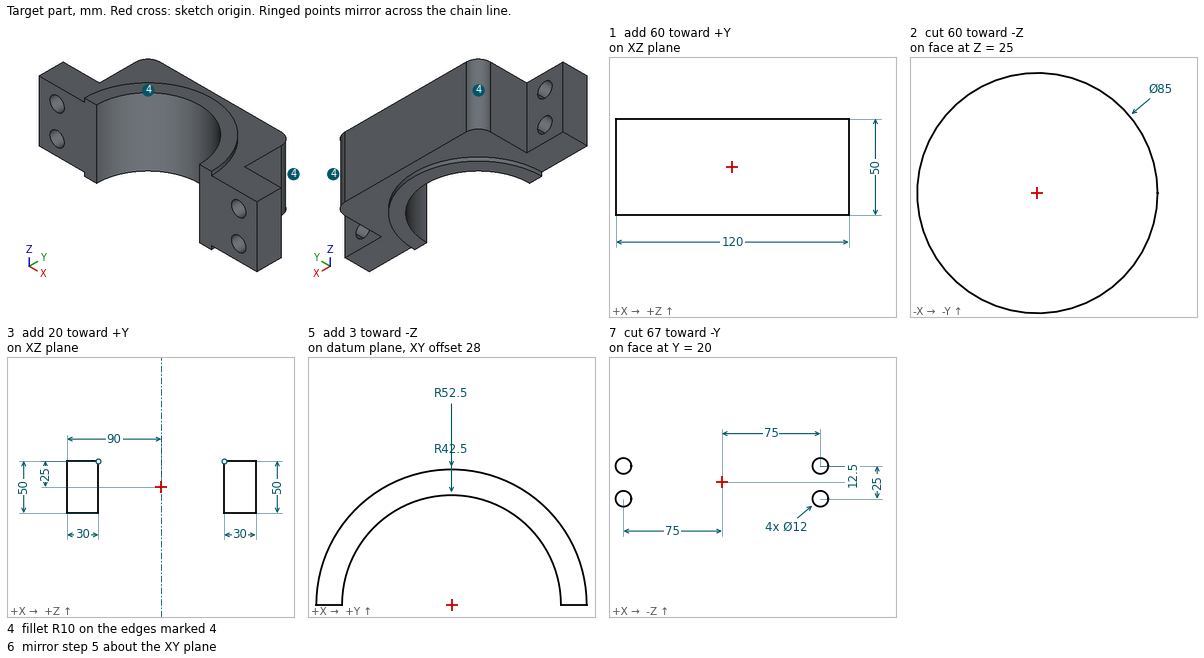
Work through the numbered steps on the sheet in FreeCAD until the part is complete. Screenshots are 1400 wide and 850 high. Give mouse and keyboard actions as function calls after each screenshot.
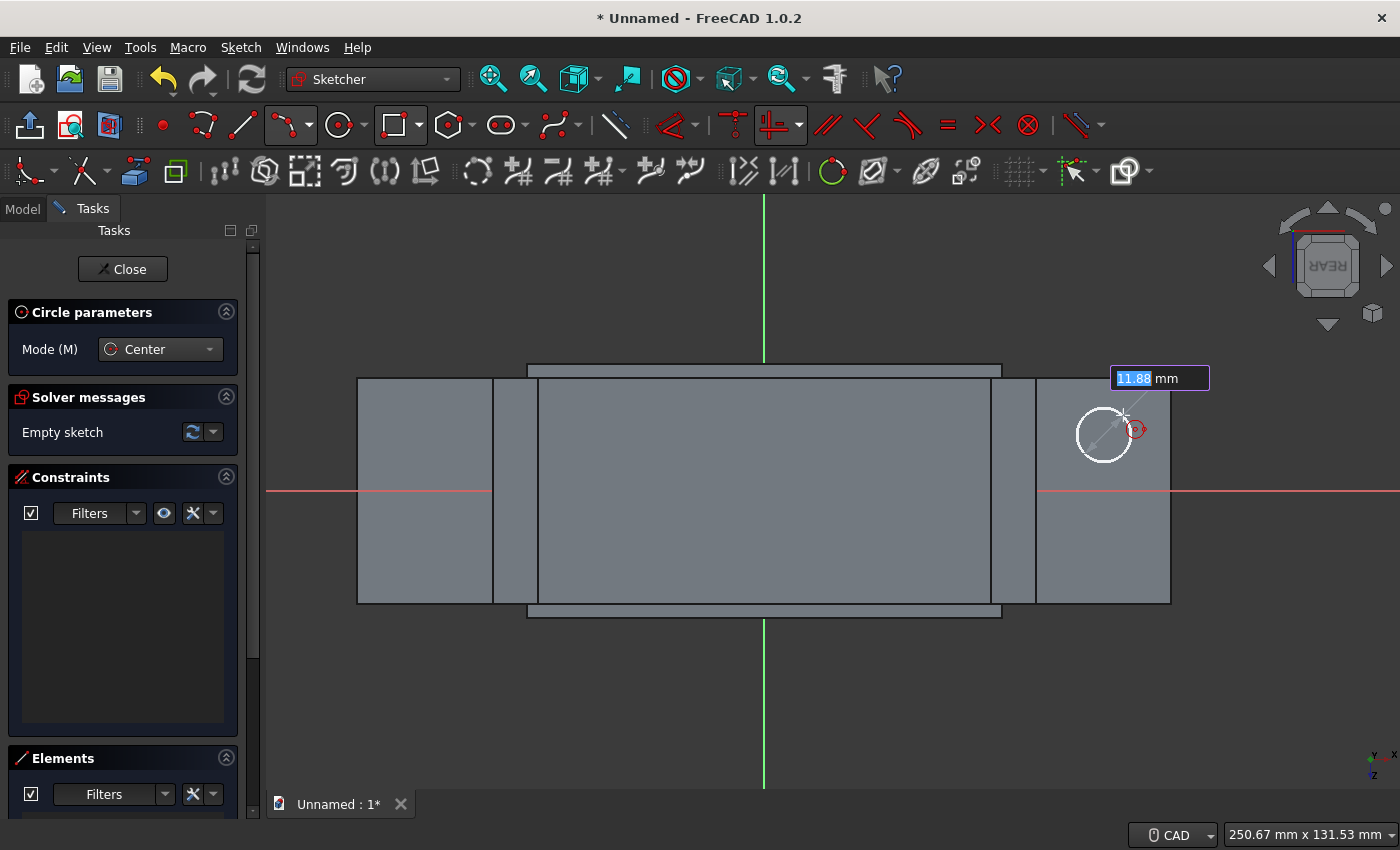
text(12)
key(Return)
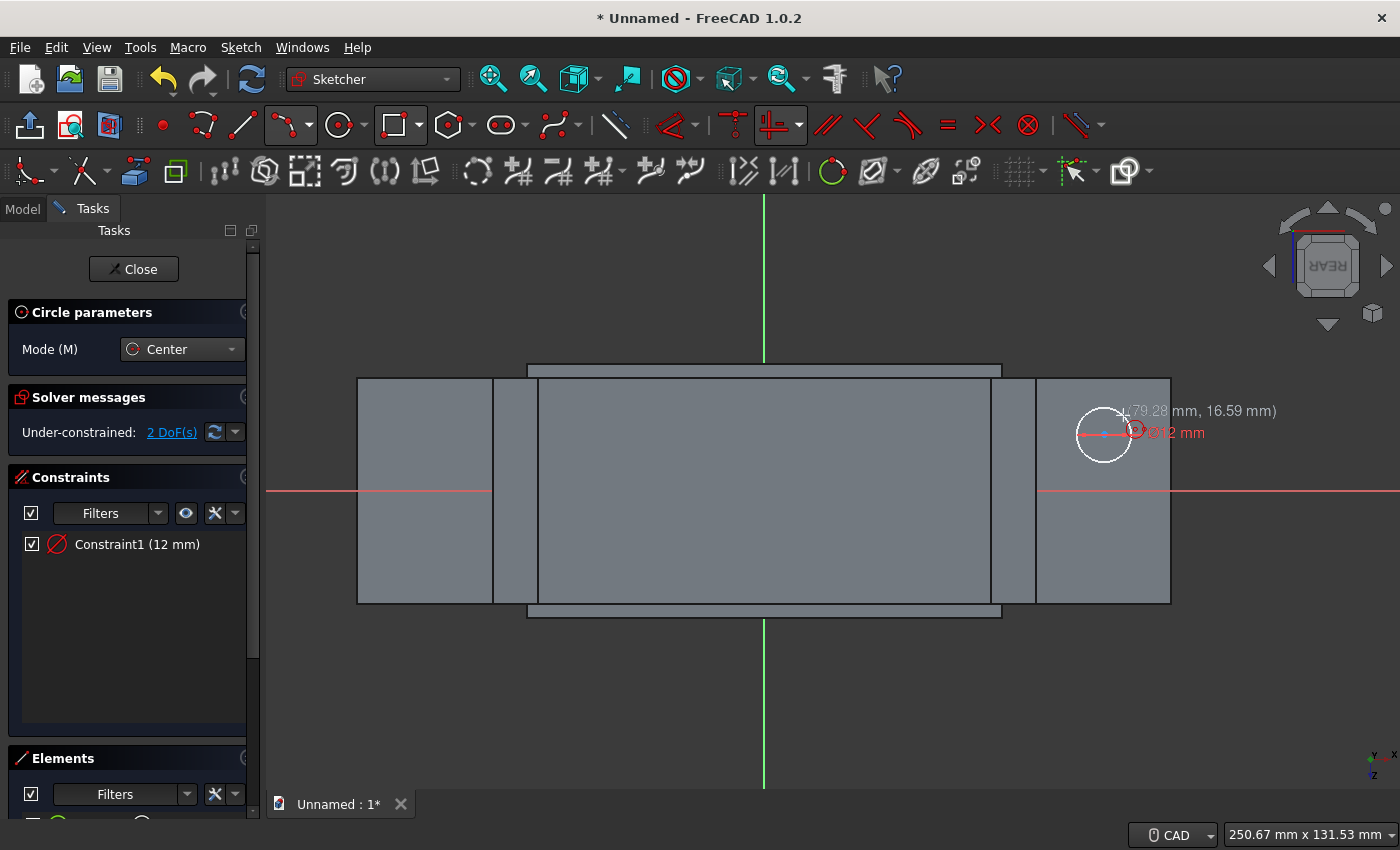
click(1104, 548)
move(1123, 528)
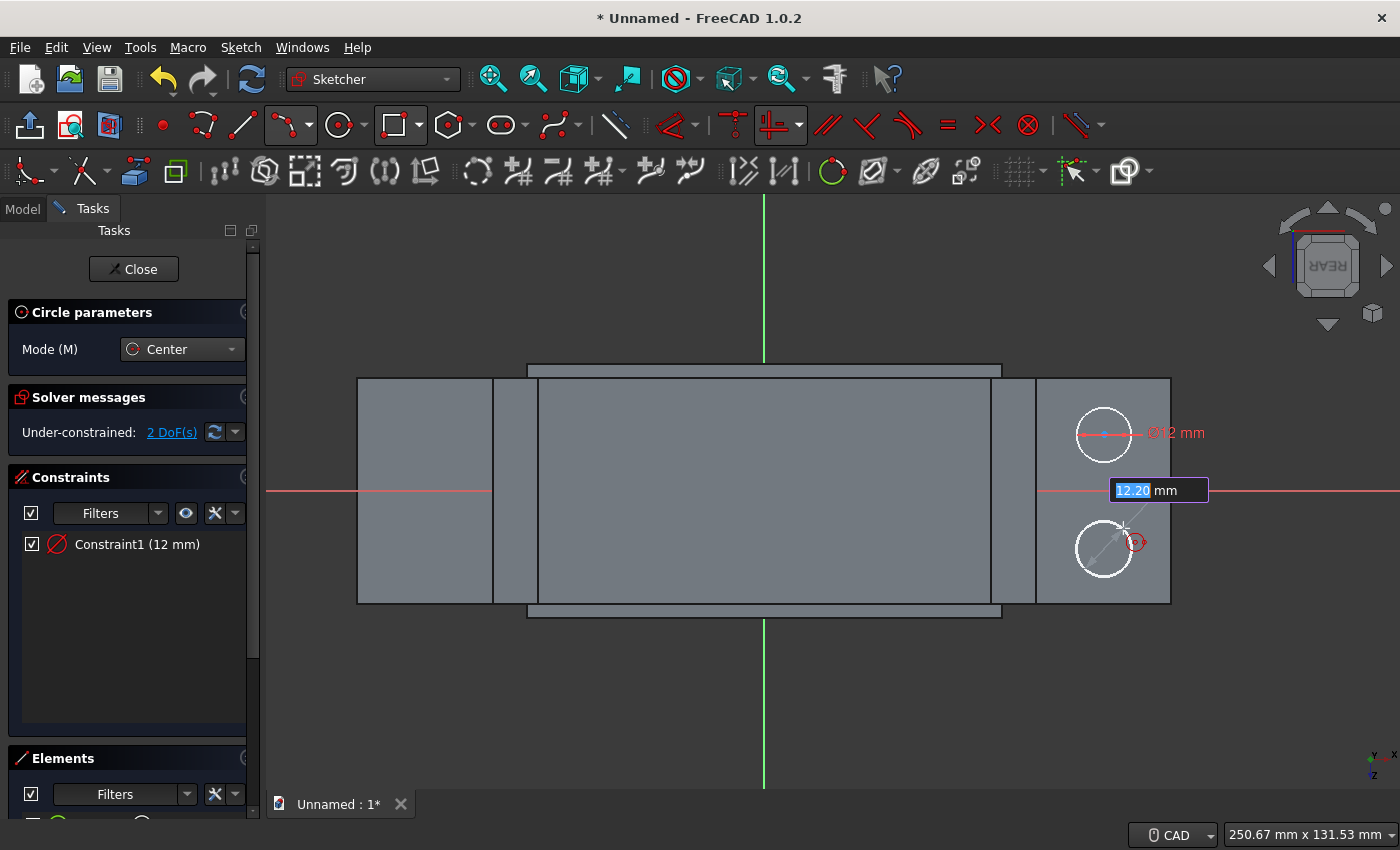
text(12)
key(Return)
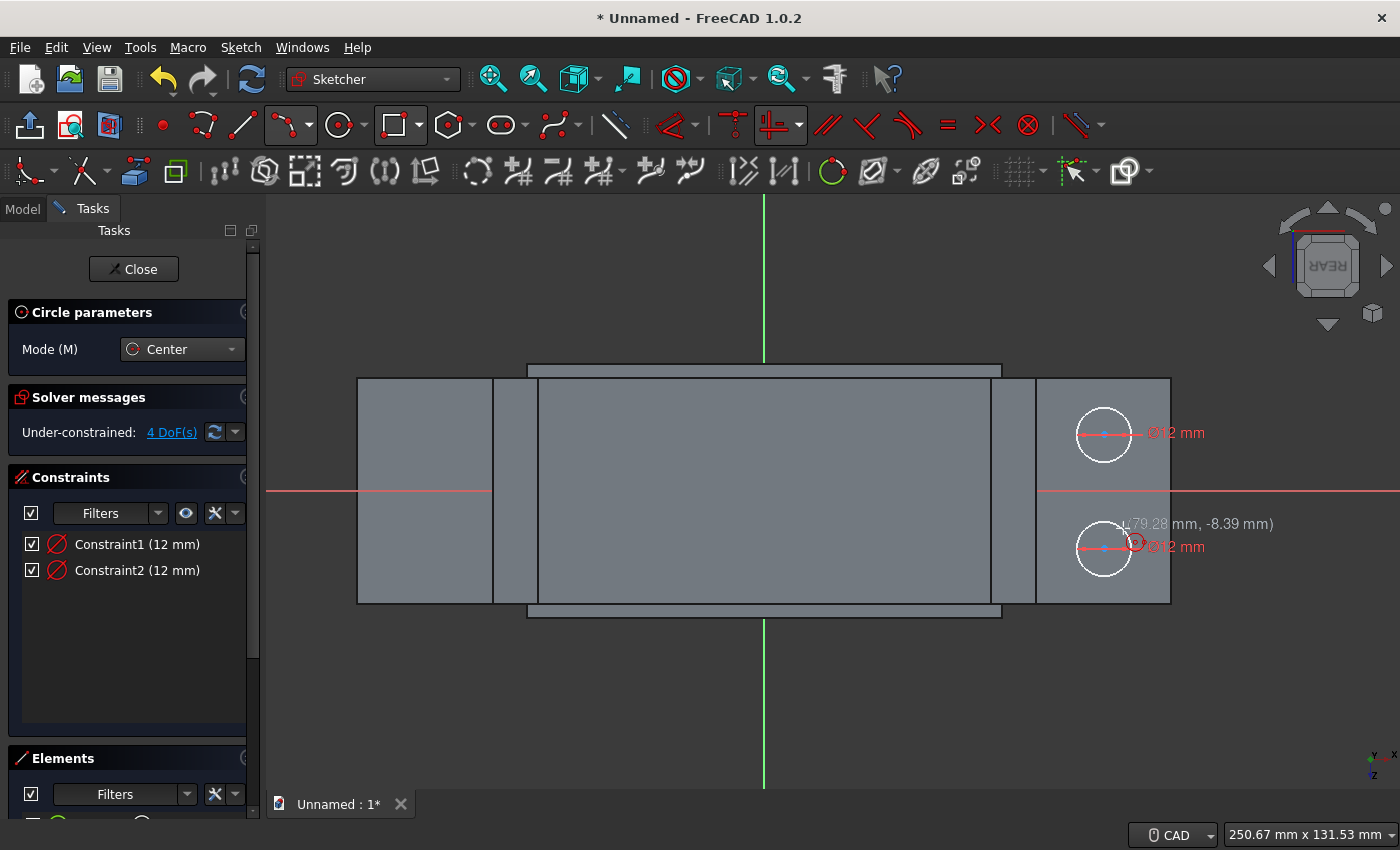
click(425, 548)
move(444, 528)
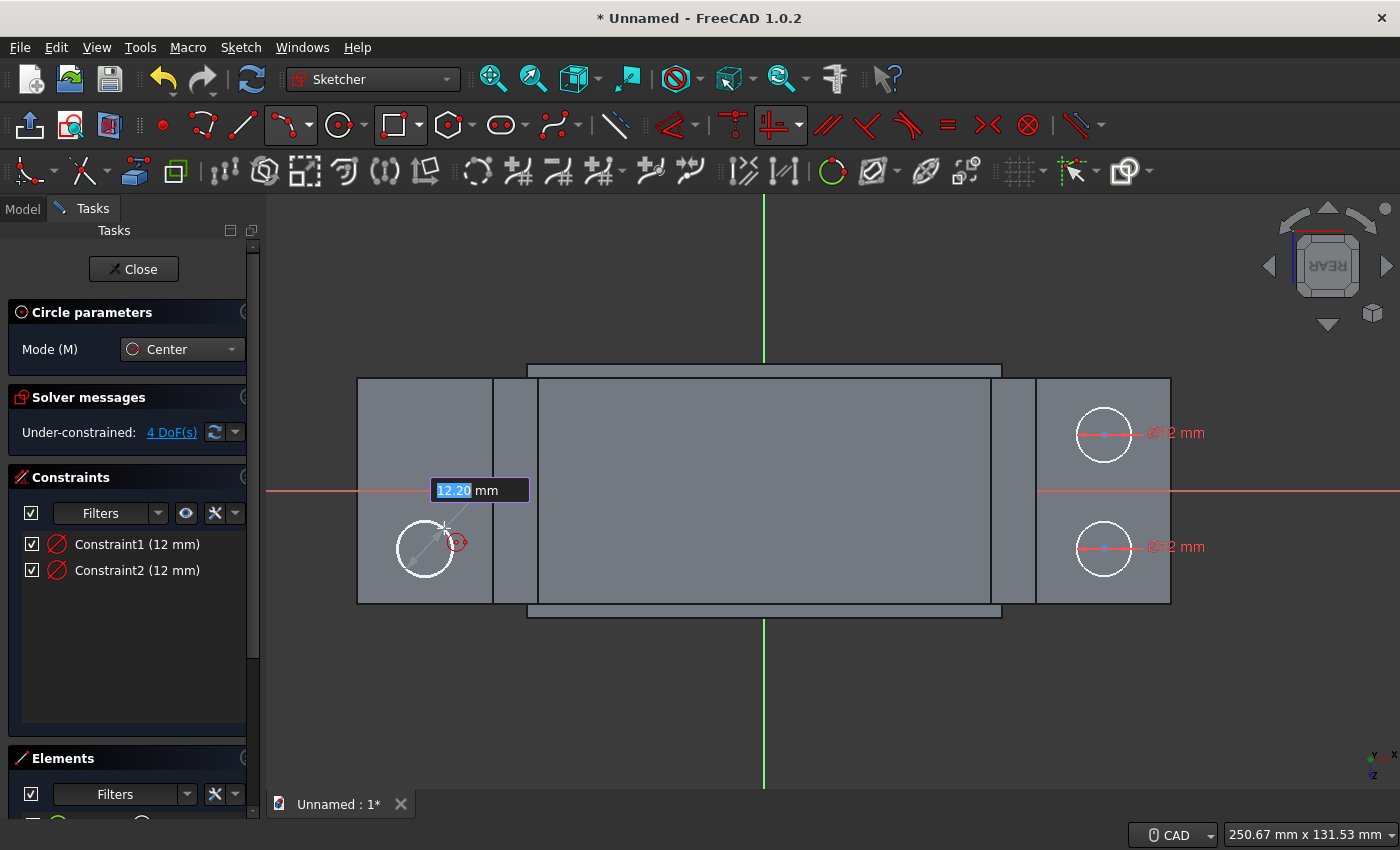
text(12)
key(Return)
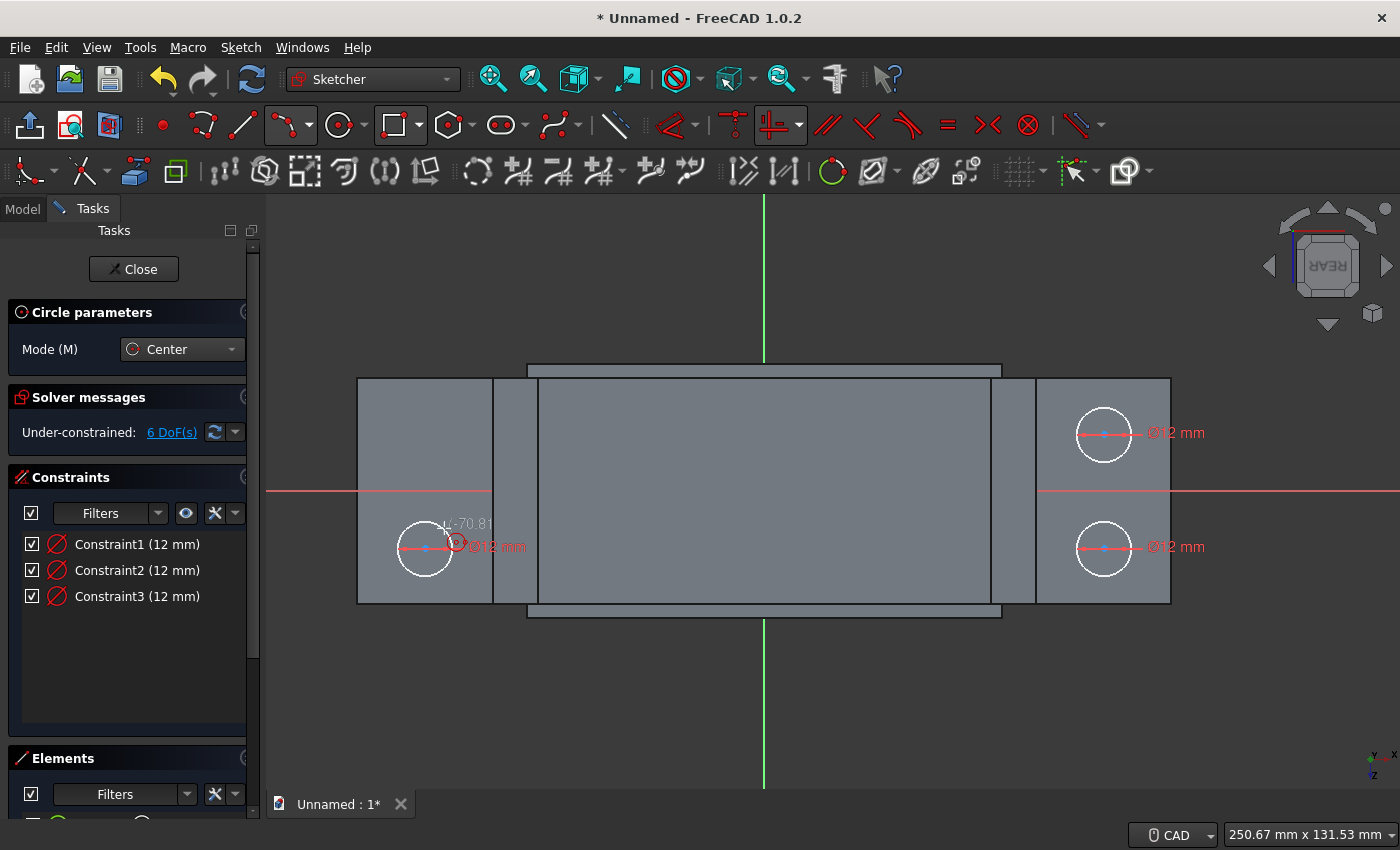
click(425, 434)
move(444, 415)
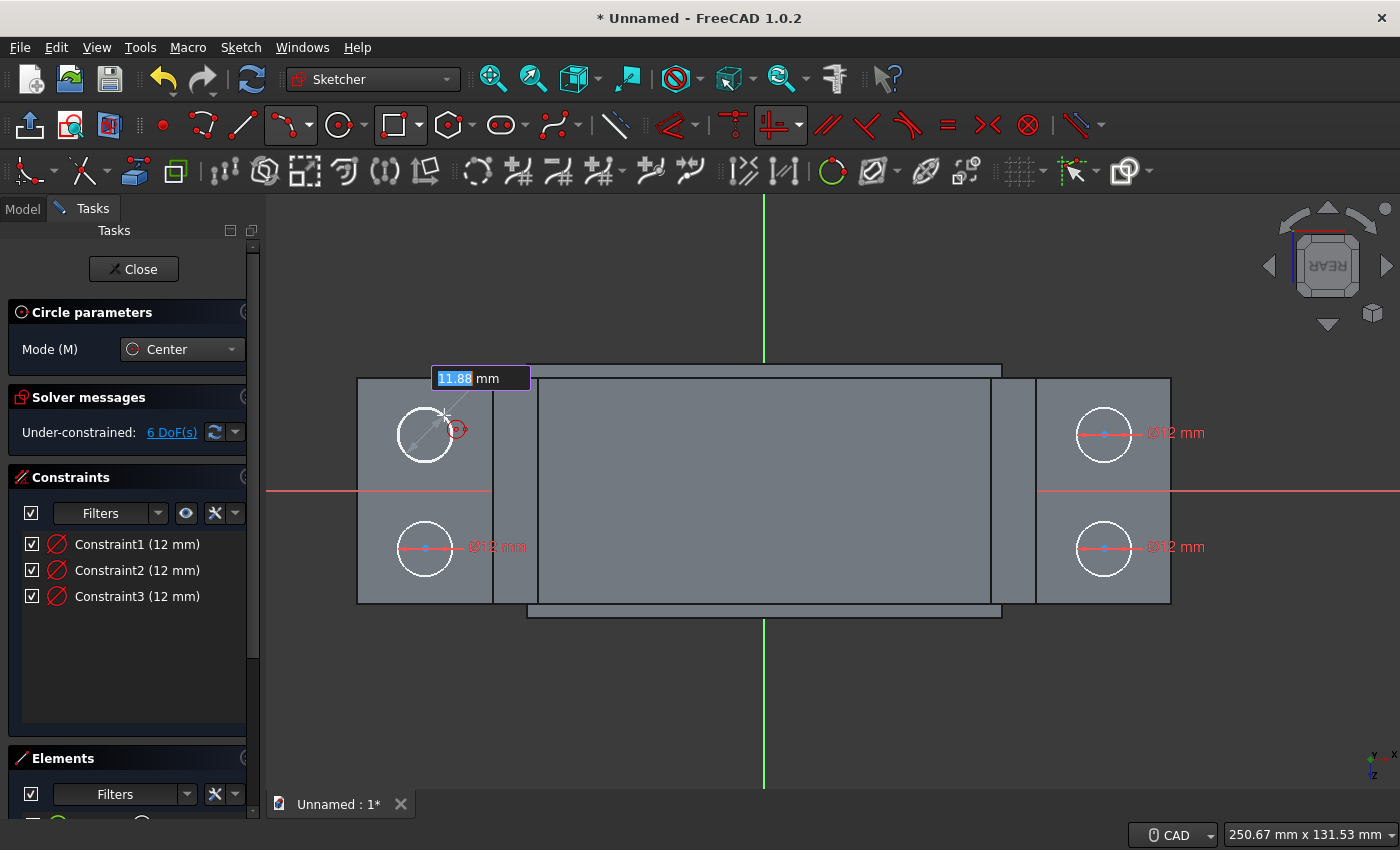
text(12)
key(Return)
key(Escape)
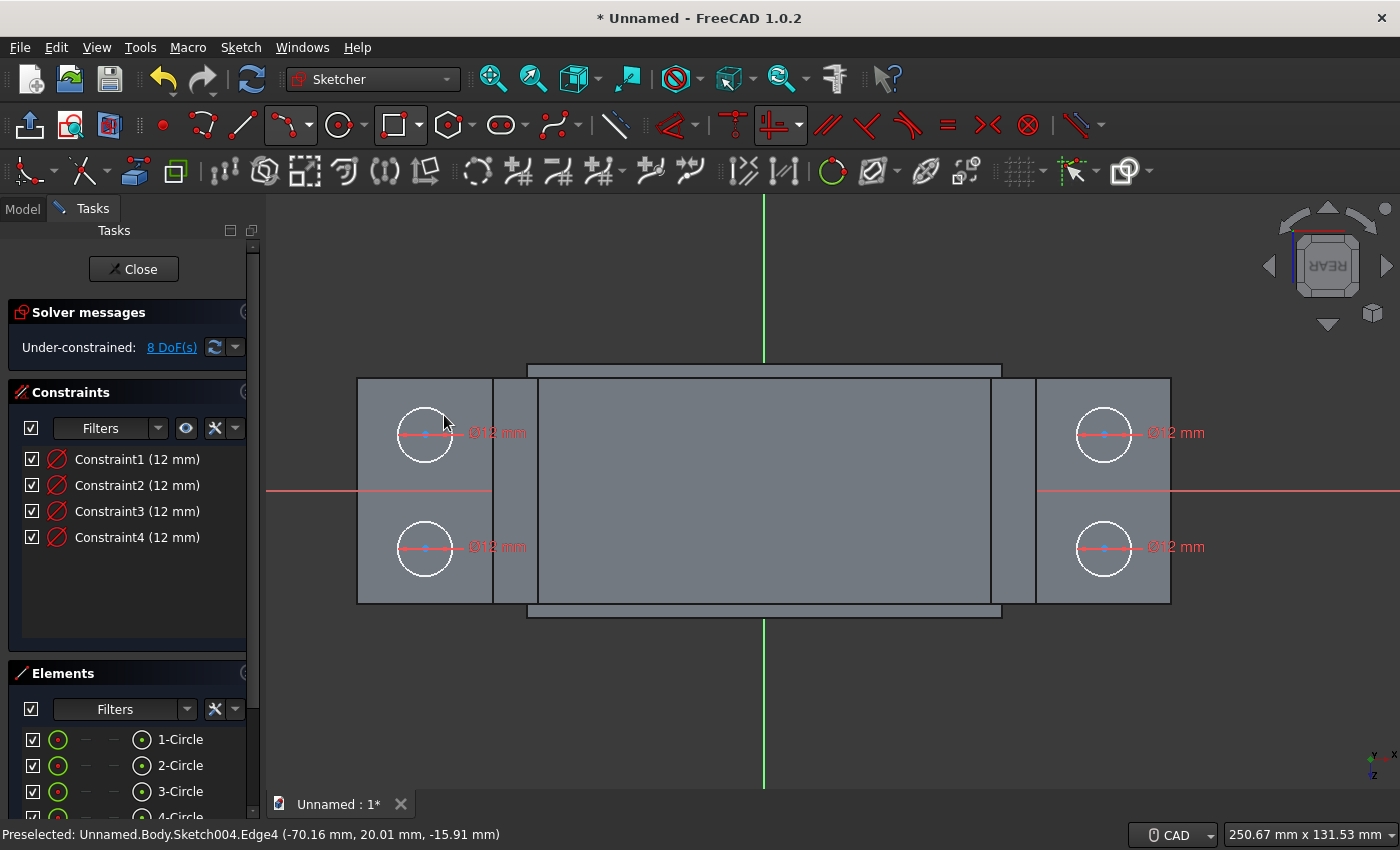
click(1104, 435)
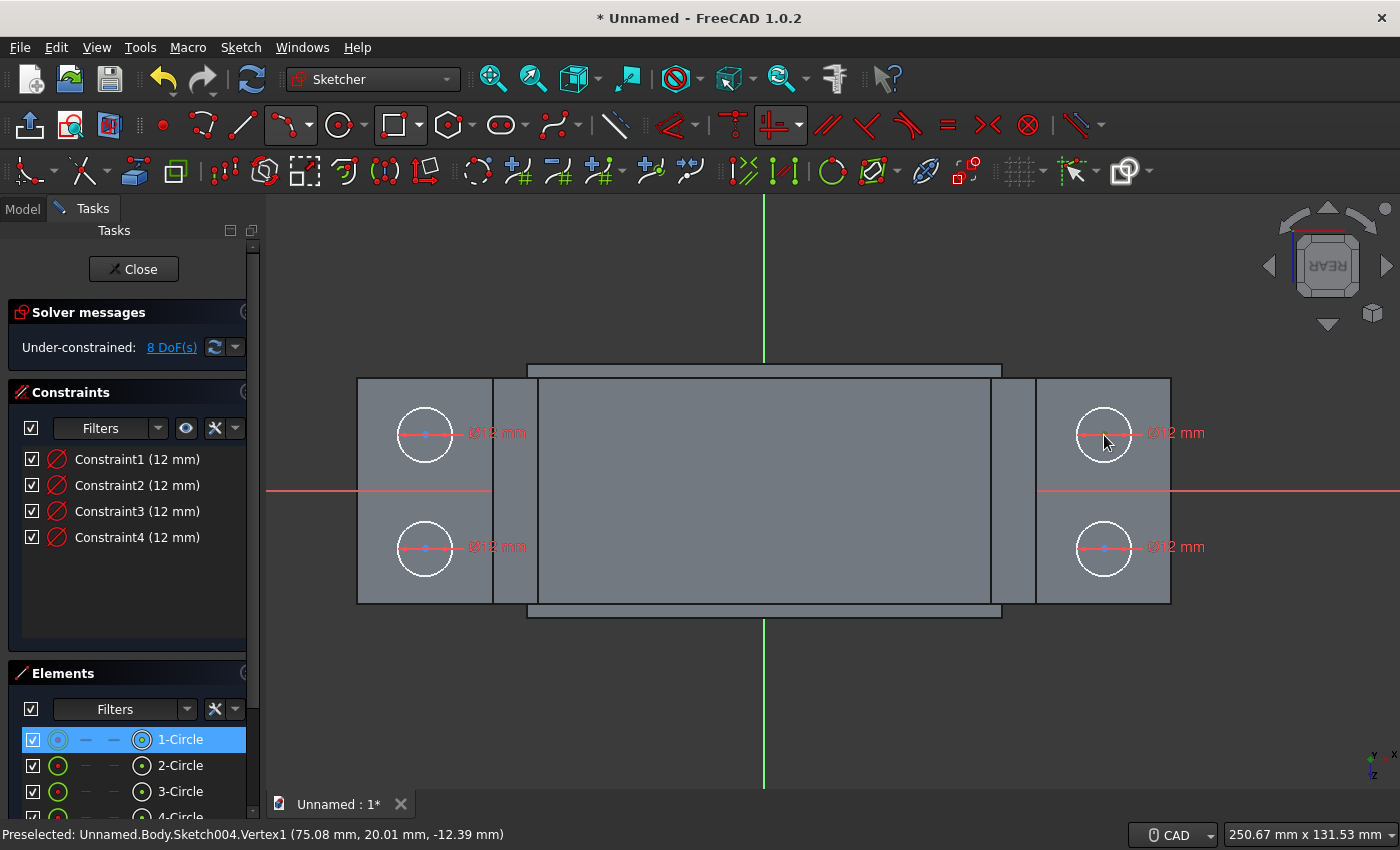
click(1104, 549)